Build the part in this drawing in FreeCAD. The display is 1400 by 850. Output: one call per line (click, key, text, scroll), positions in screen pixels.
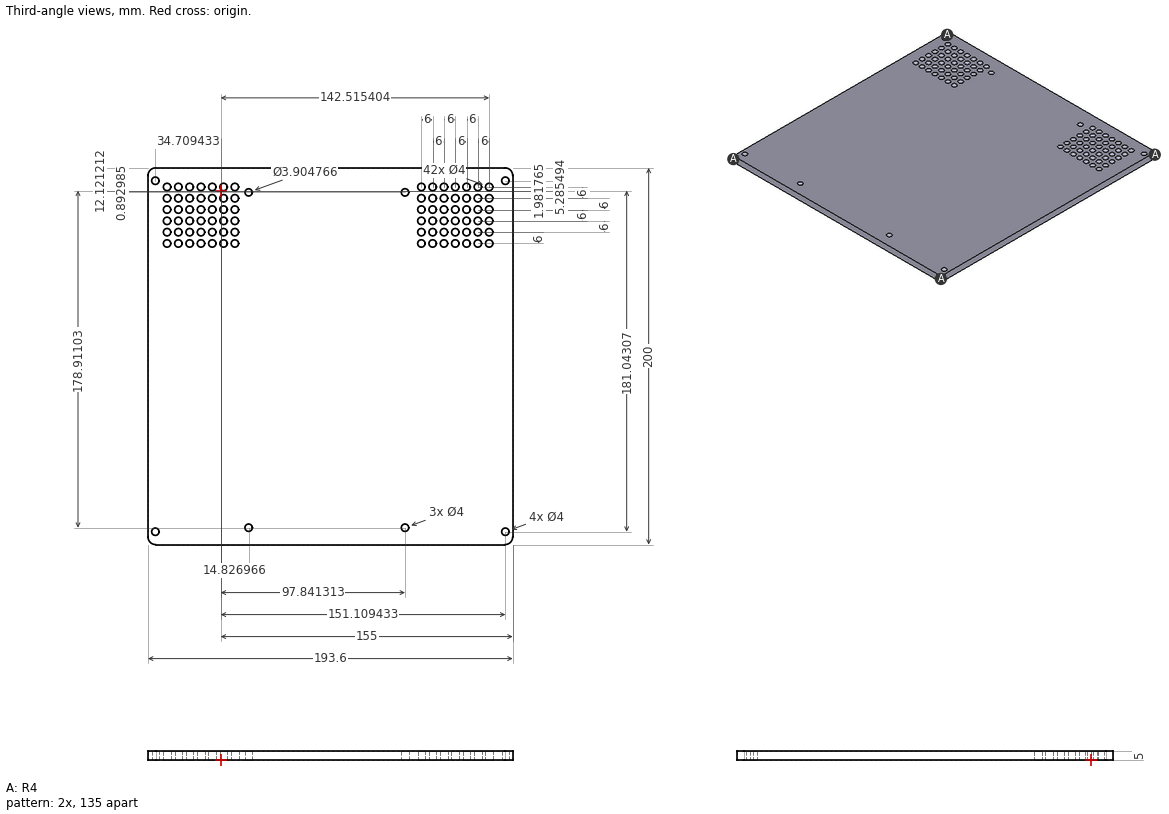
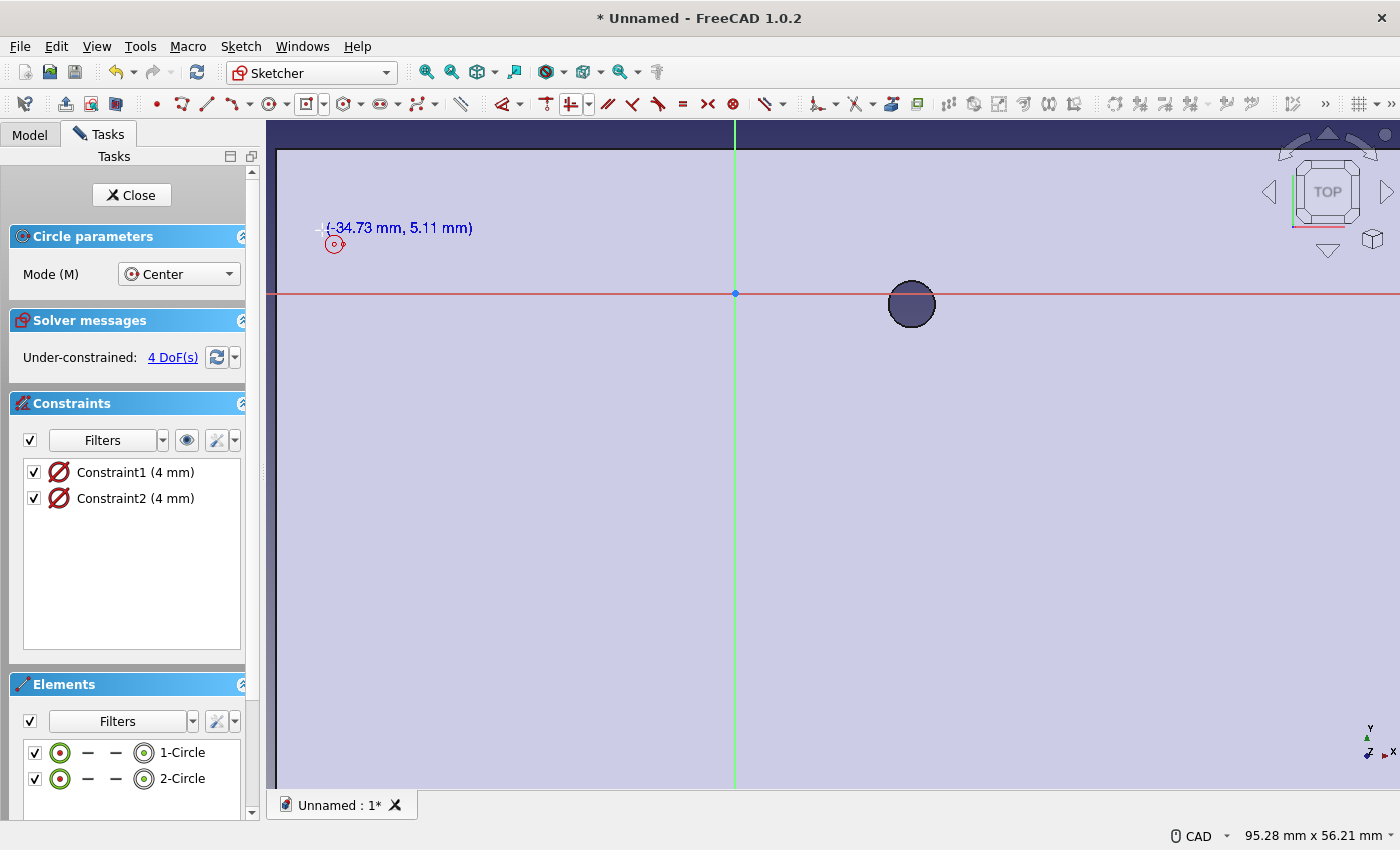
scroll(597, 231, down, 8)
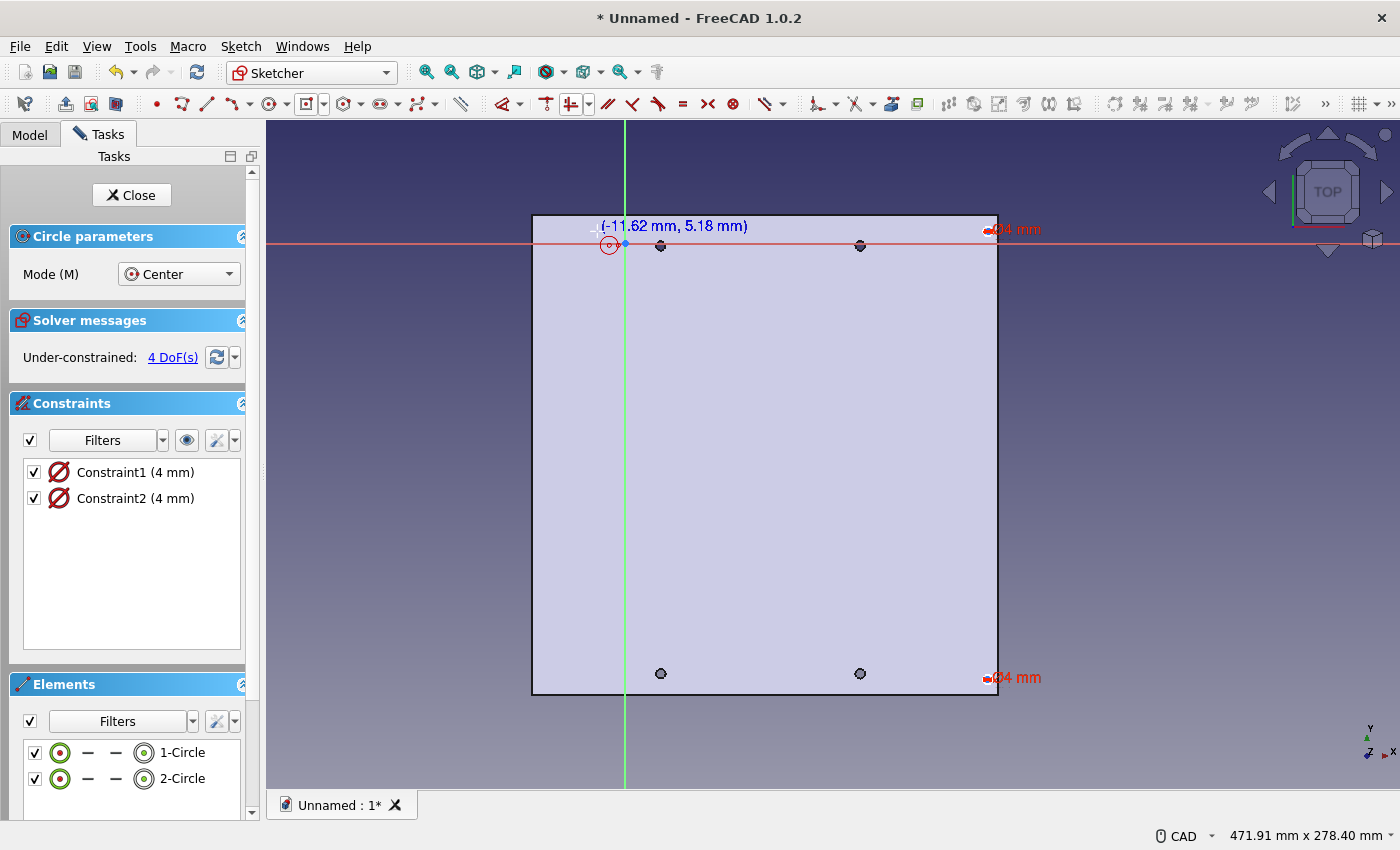
scroll(542, 231, up, 2)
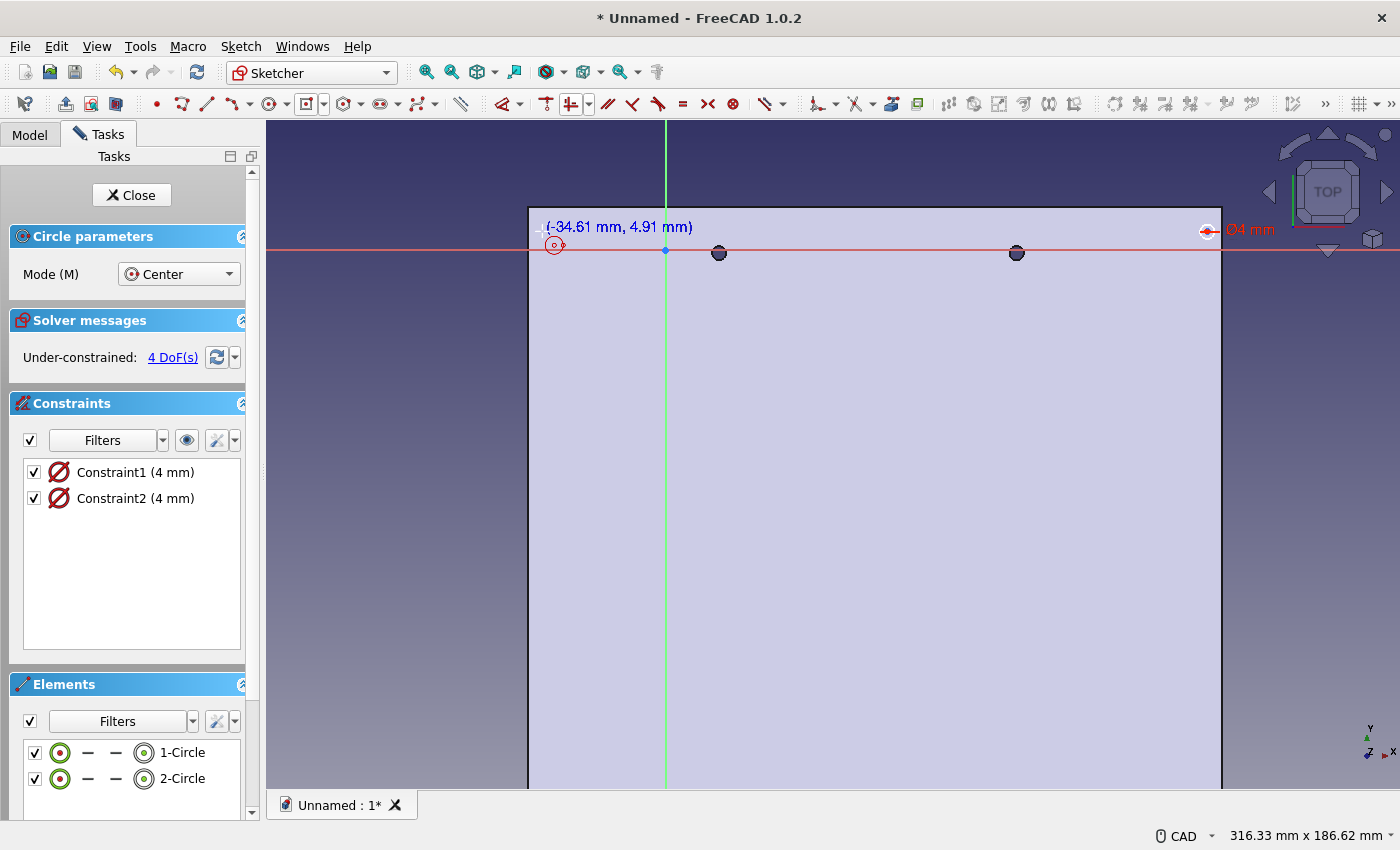
click(542, 231)
move(547, 226)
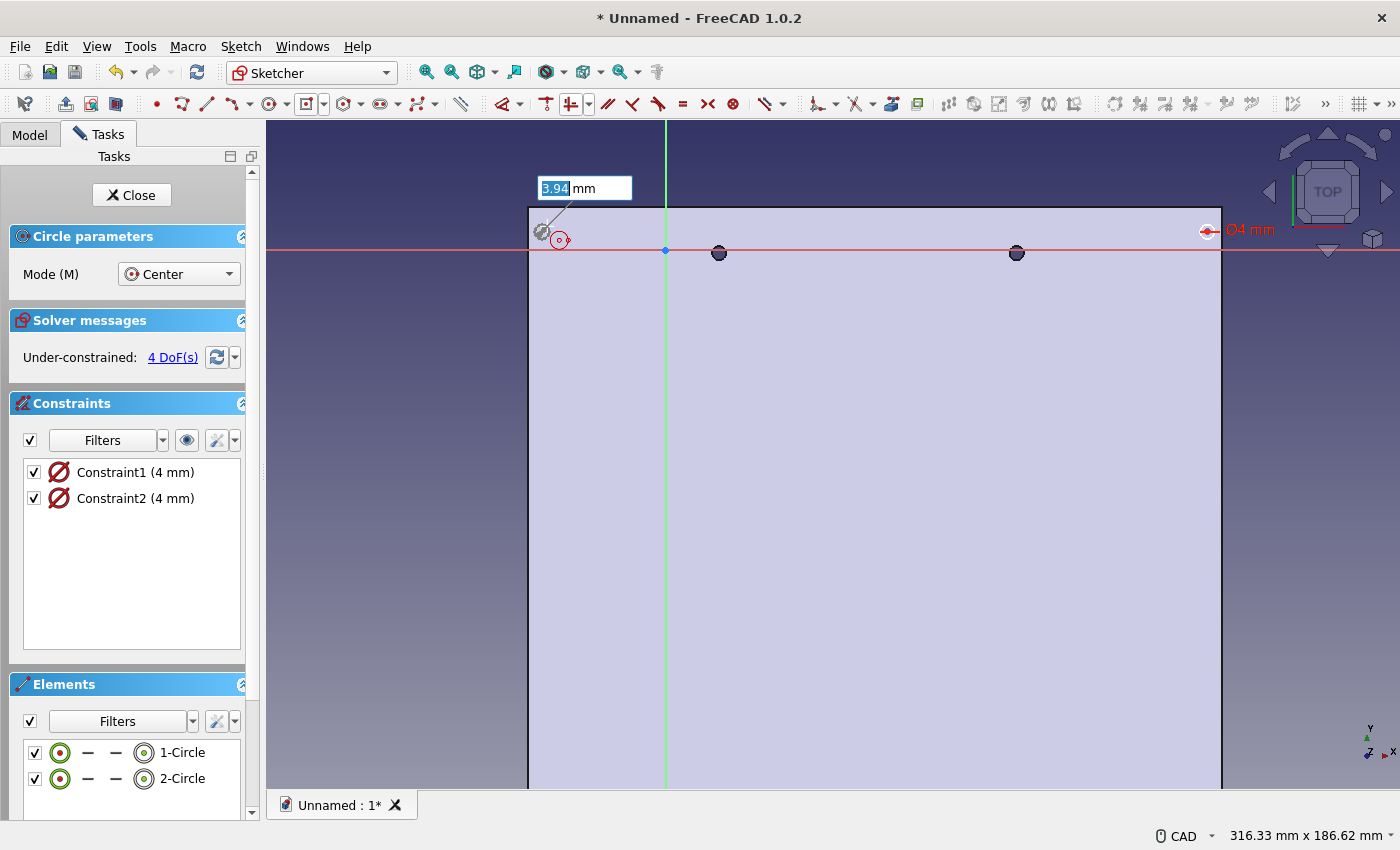
text(4)
key(Return)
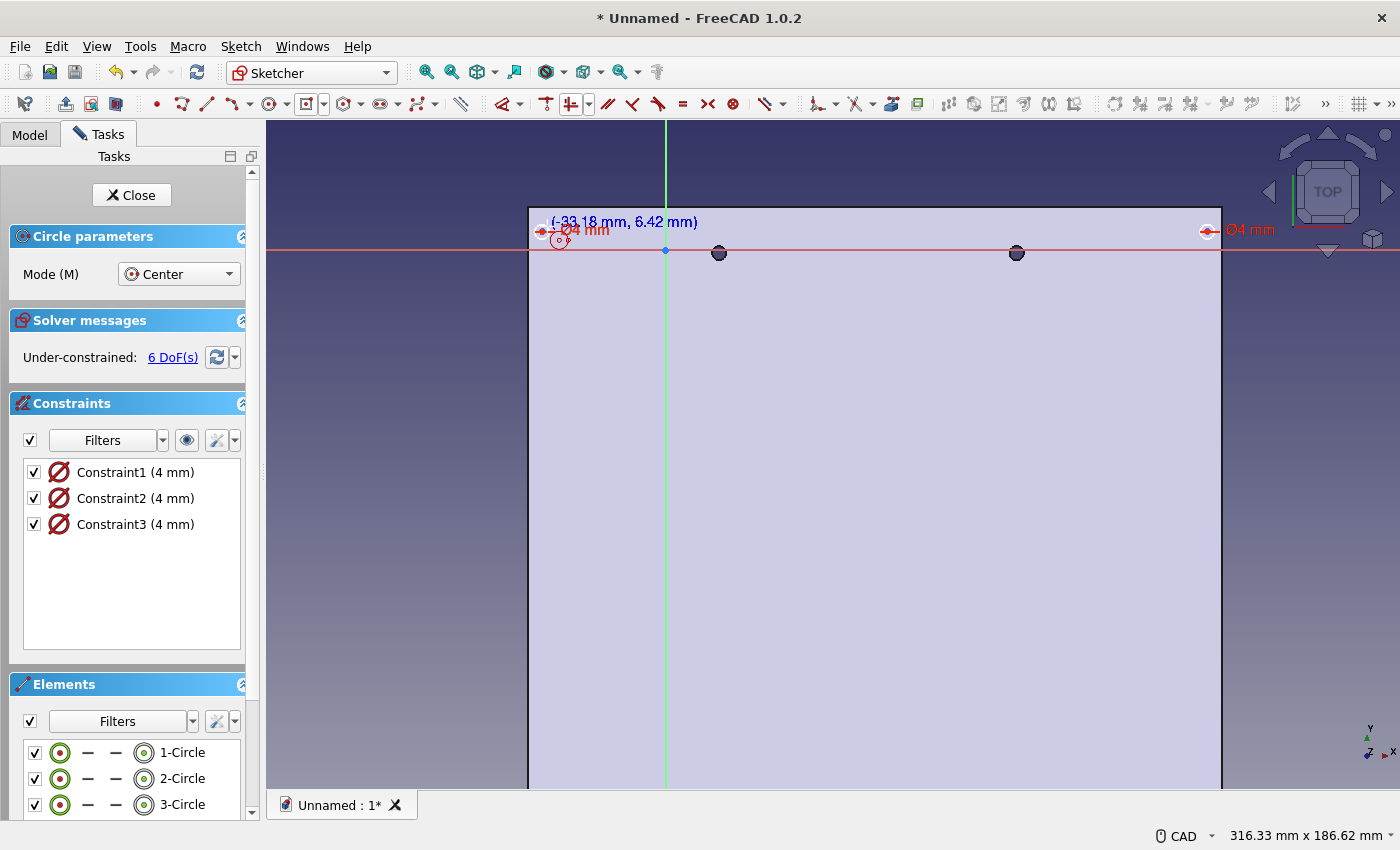
scroll(541, 230, down, 2)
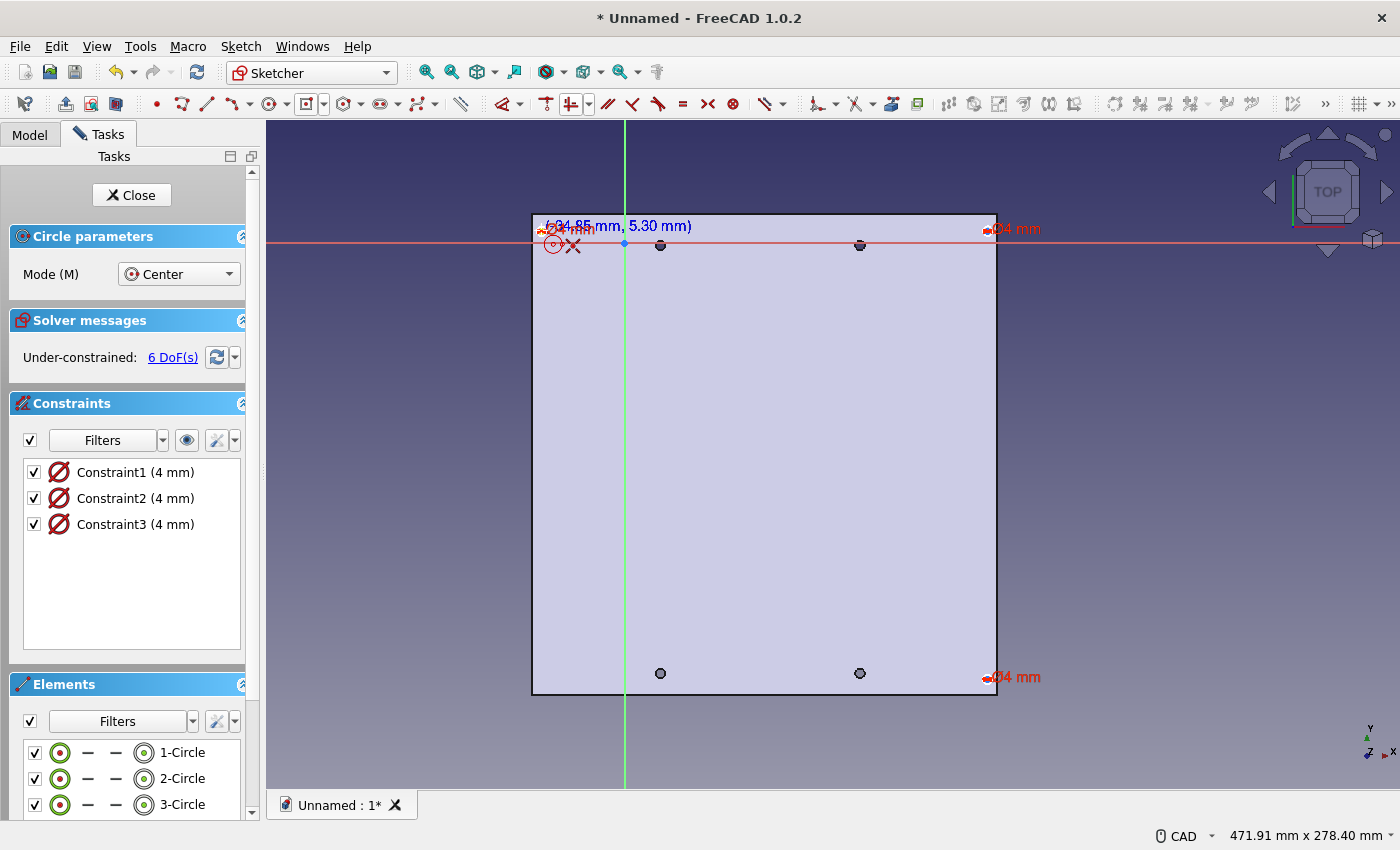
scroll(541, 679, up, 8)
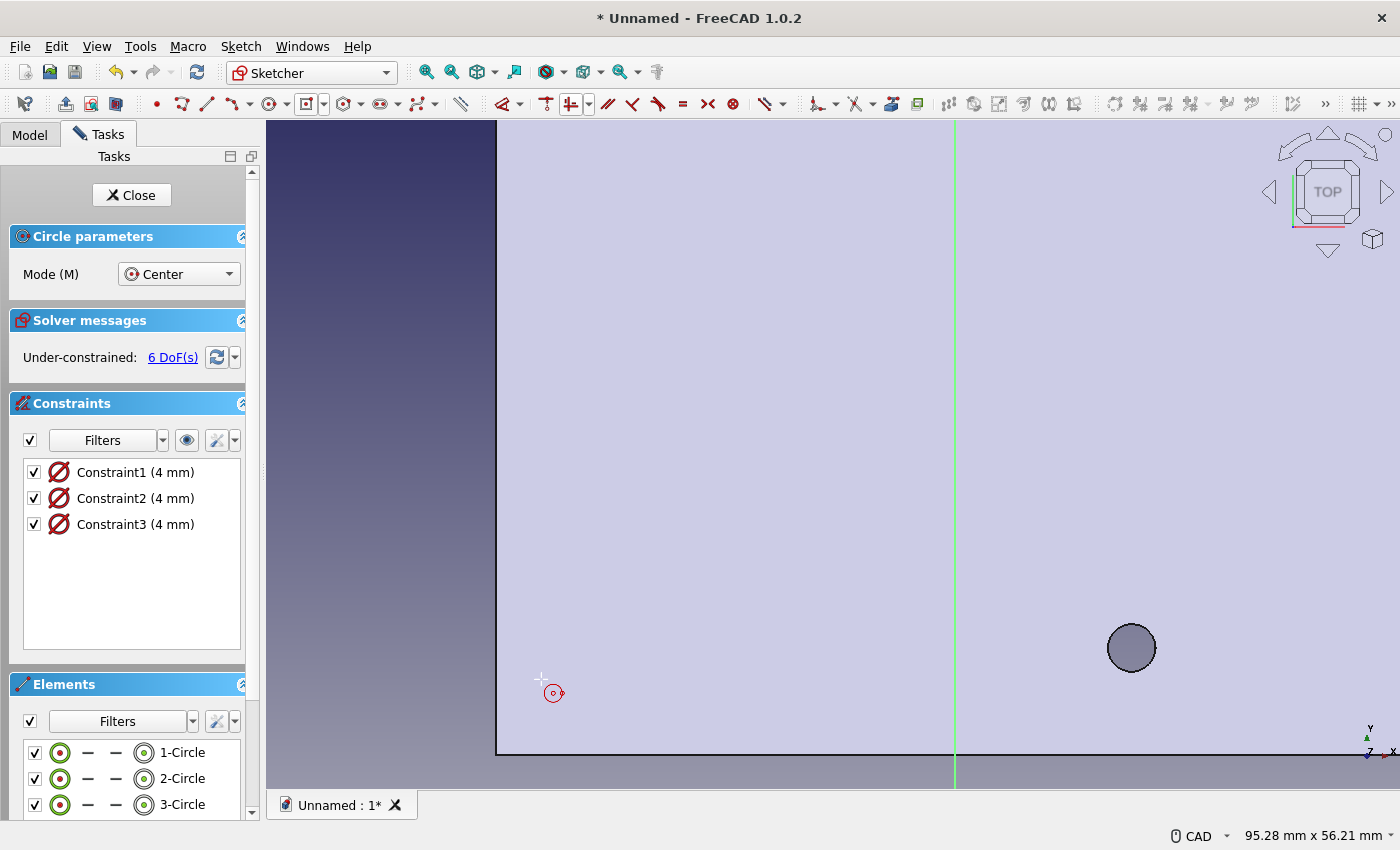
scroll(541, 680, down, 8)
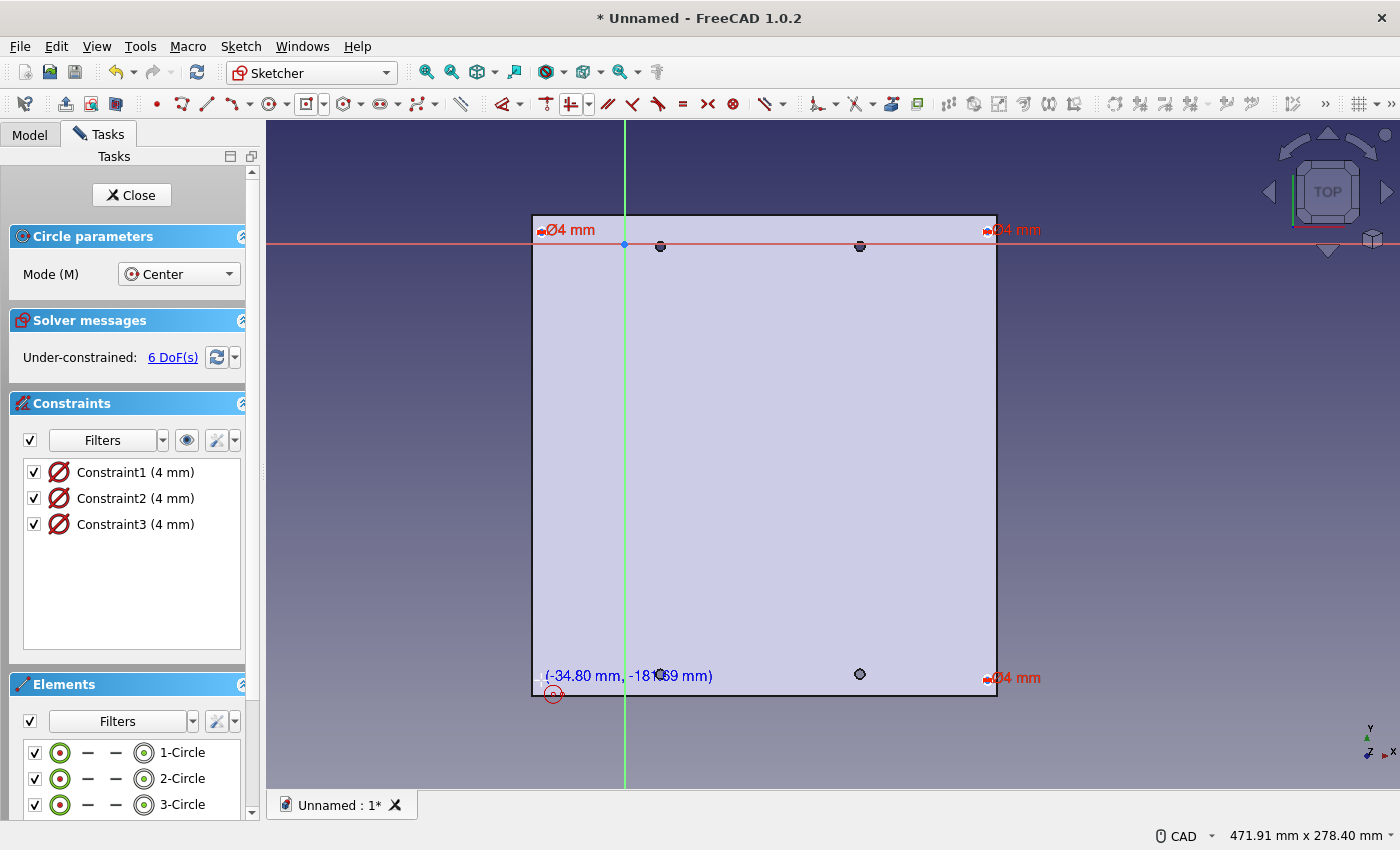
click(541, 679)
move(545, 676)